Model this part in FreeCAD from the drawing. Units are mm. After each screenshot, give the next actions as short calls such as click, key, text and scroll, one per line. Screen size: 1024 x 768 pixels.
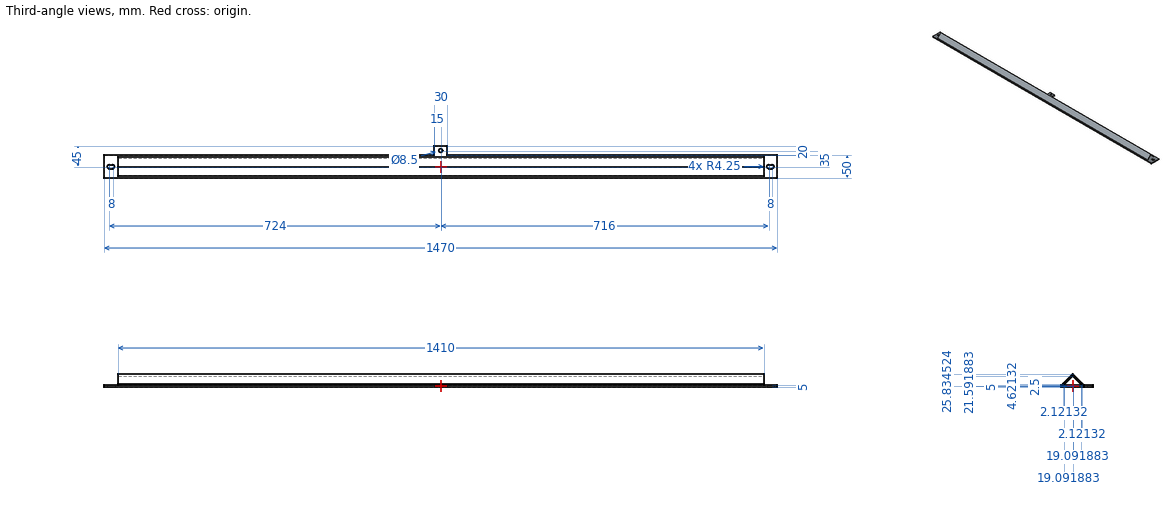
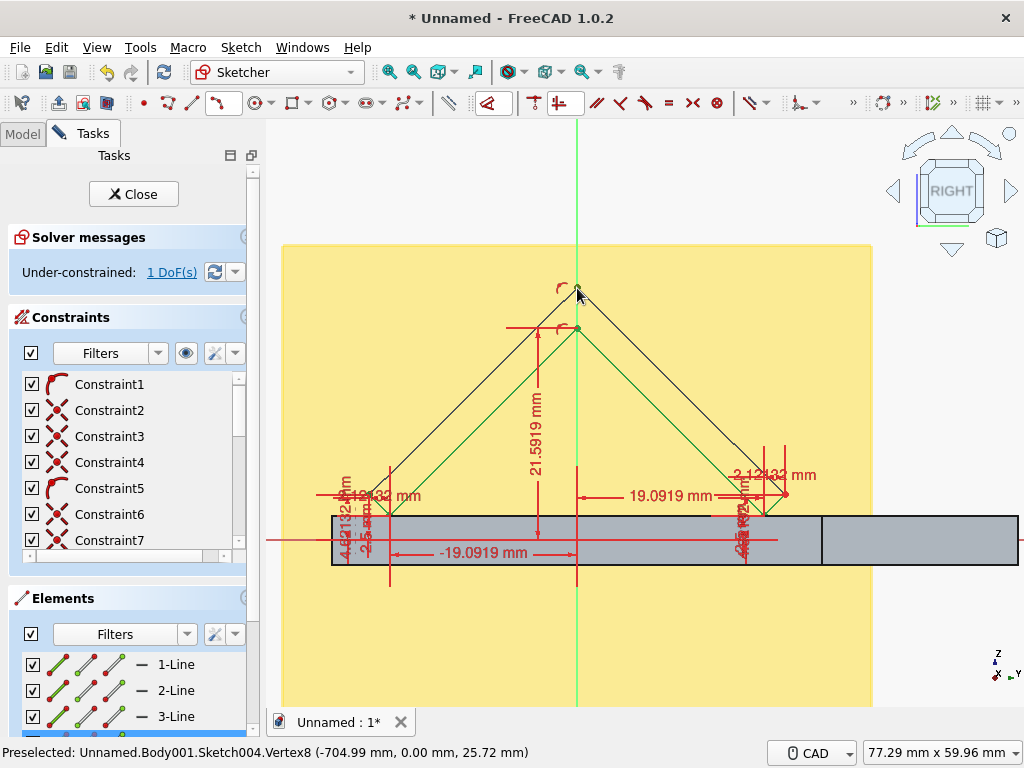
key(i)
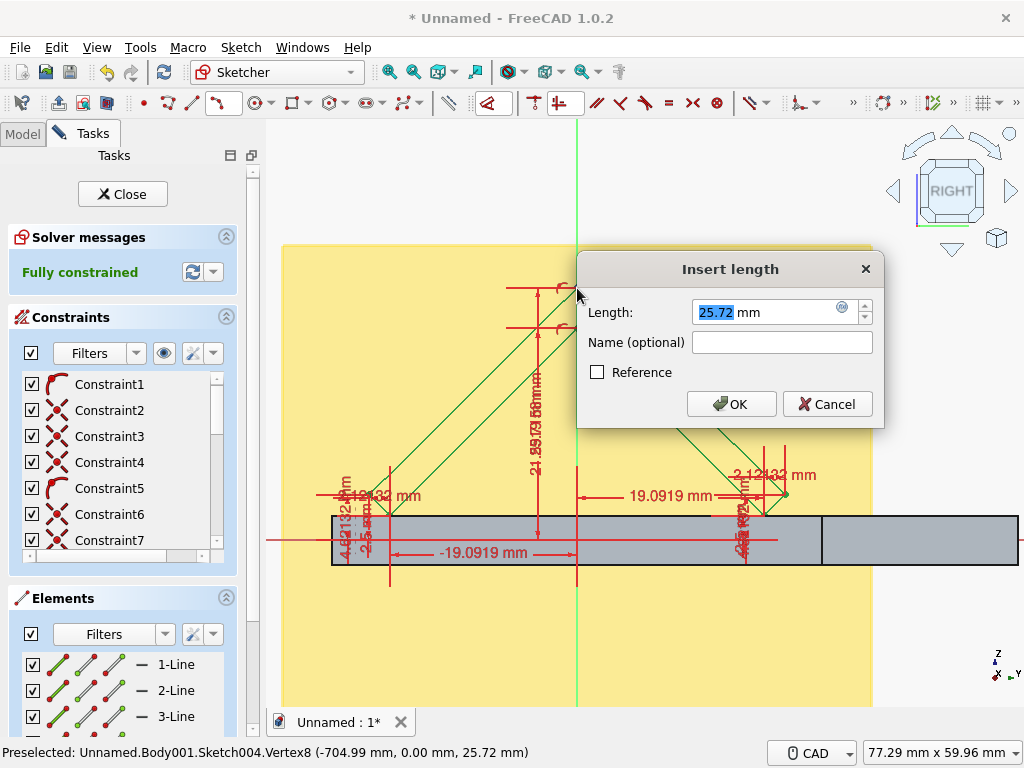
text(25.834524)
key(Return)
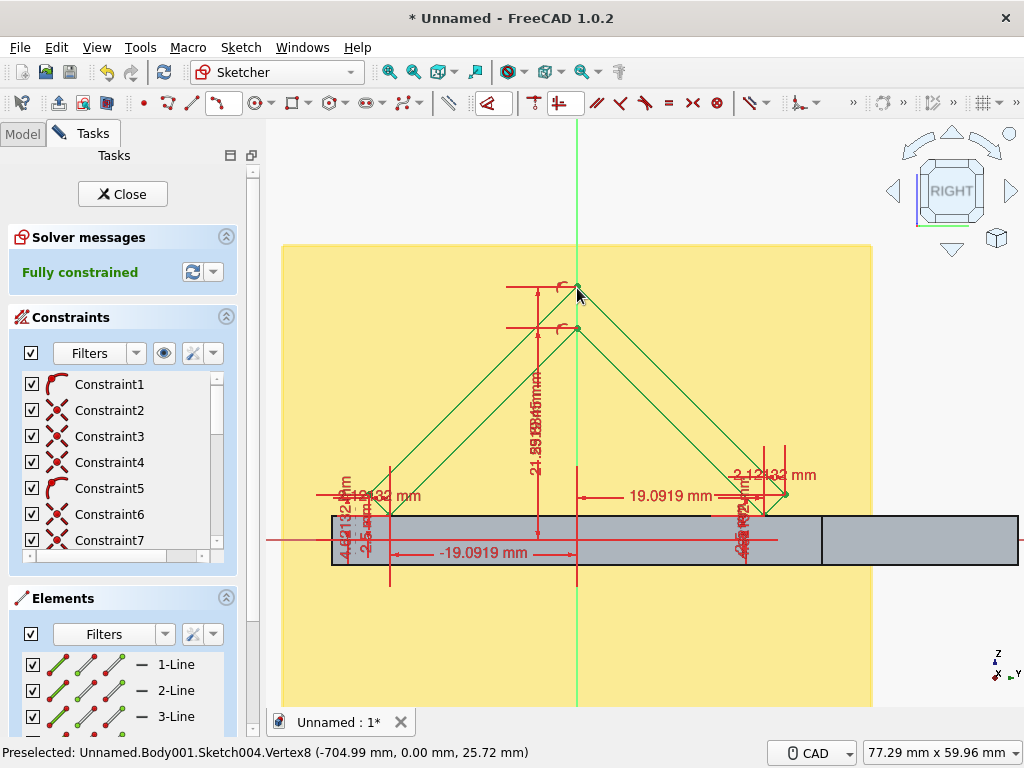
click(123, 194)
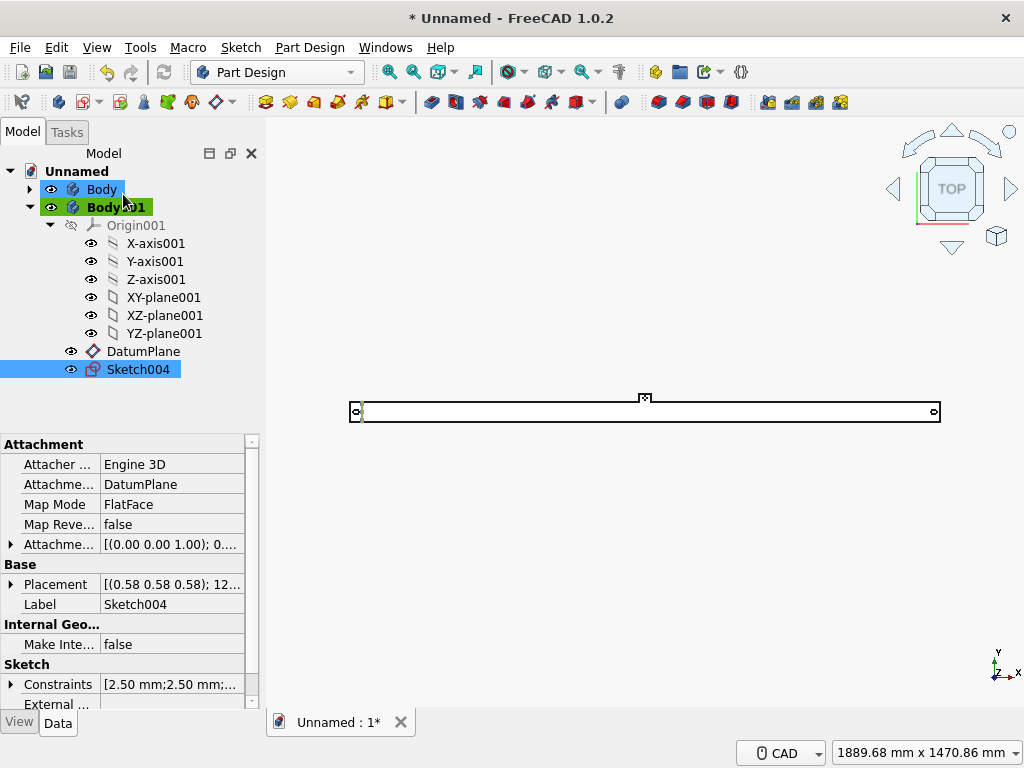
click(266, 102)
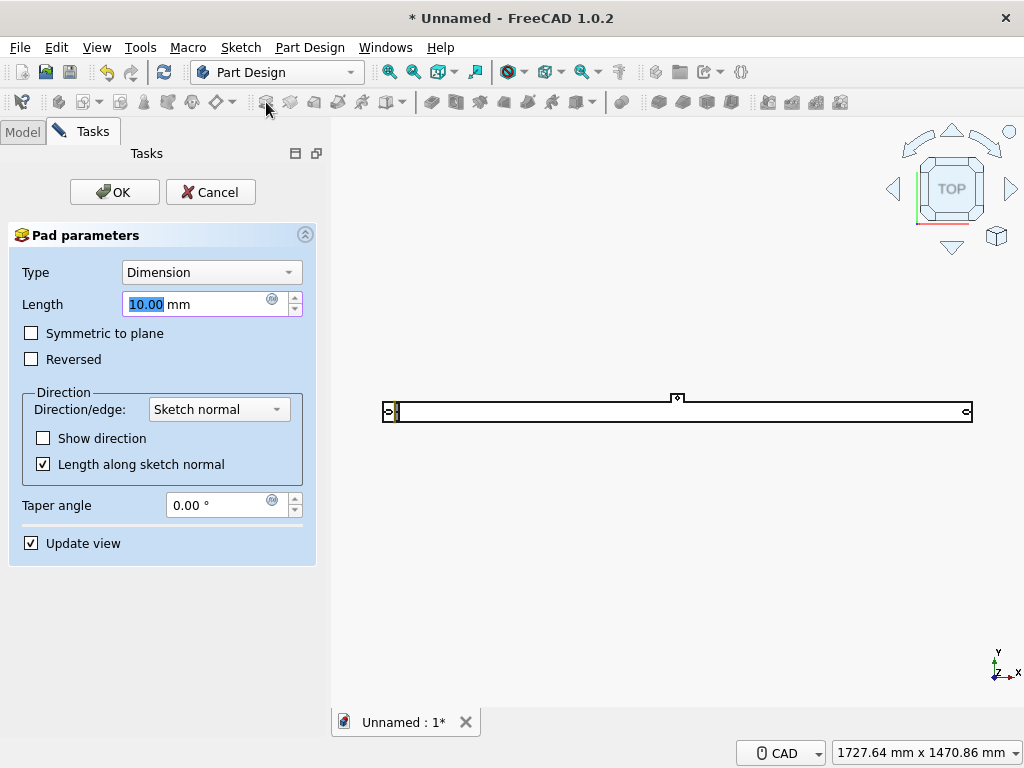
text(1410)
key(Tab)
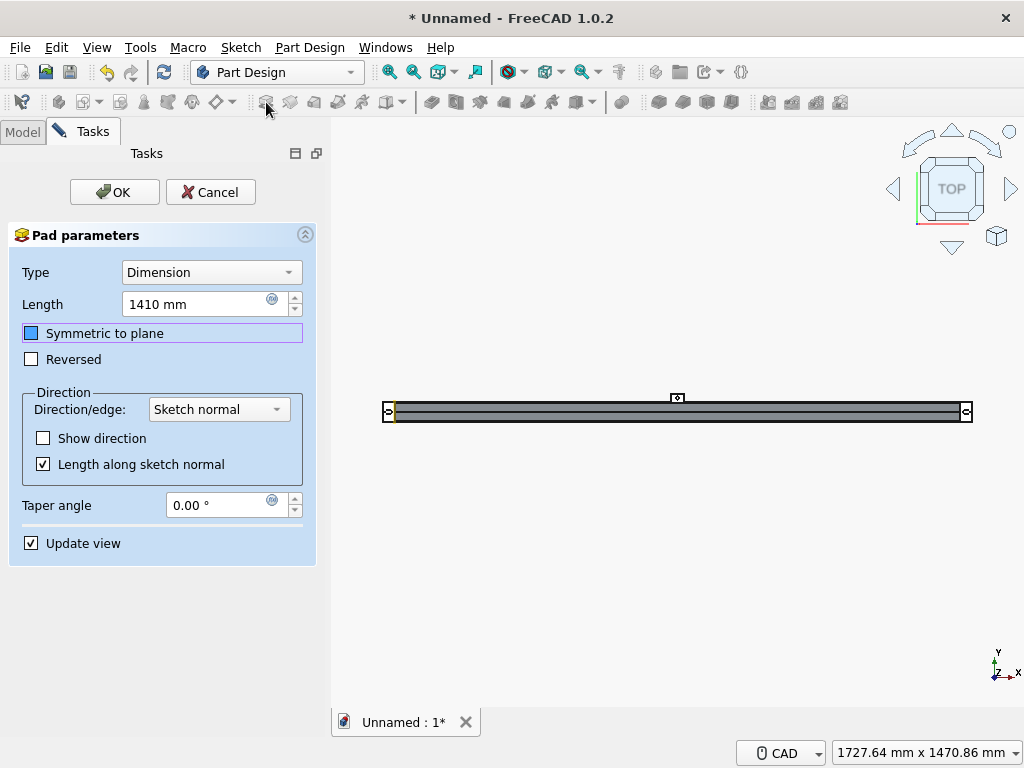
click(115, 192)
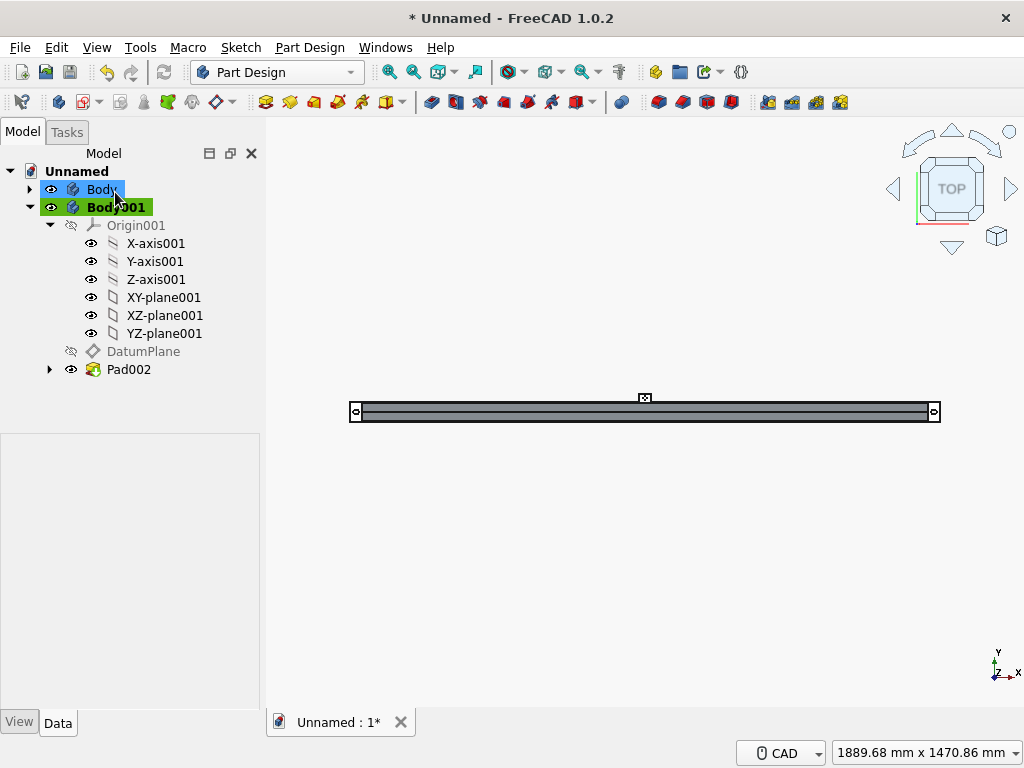
key(0)